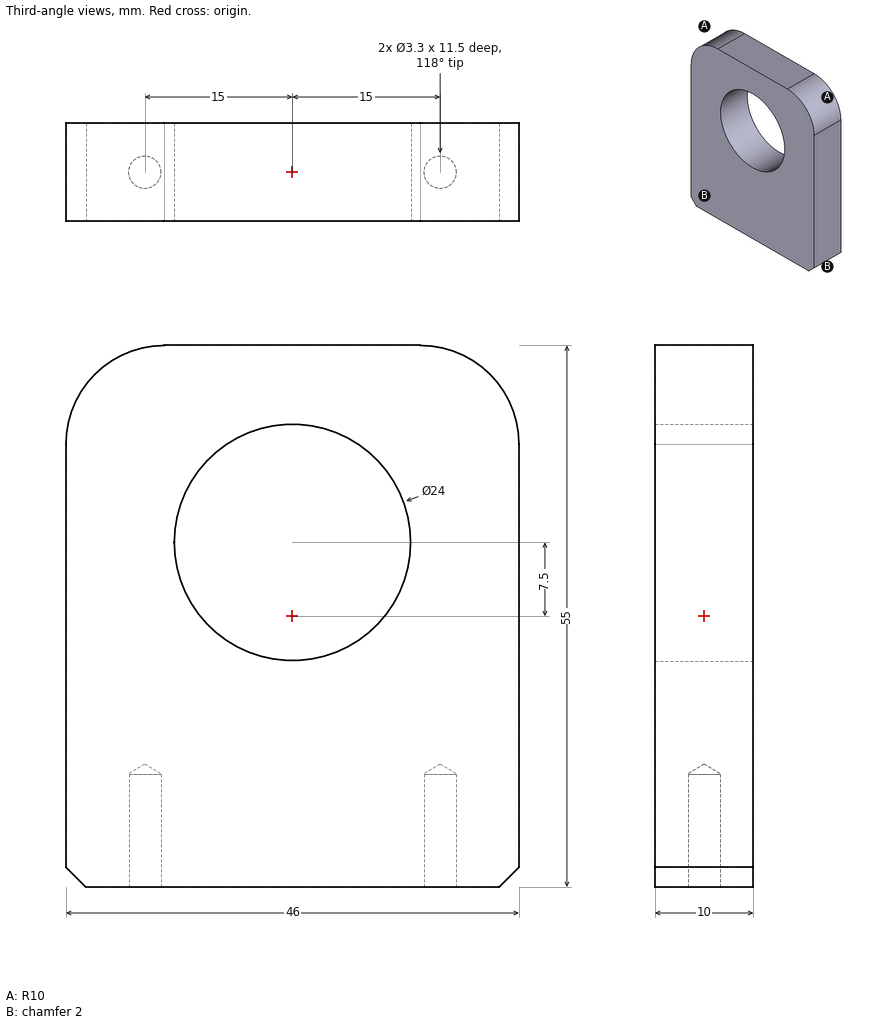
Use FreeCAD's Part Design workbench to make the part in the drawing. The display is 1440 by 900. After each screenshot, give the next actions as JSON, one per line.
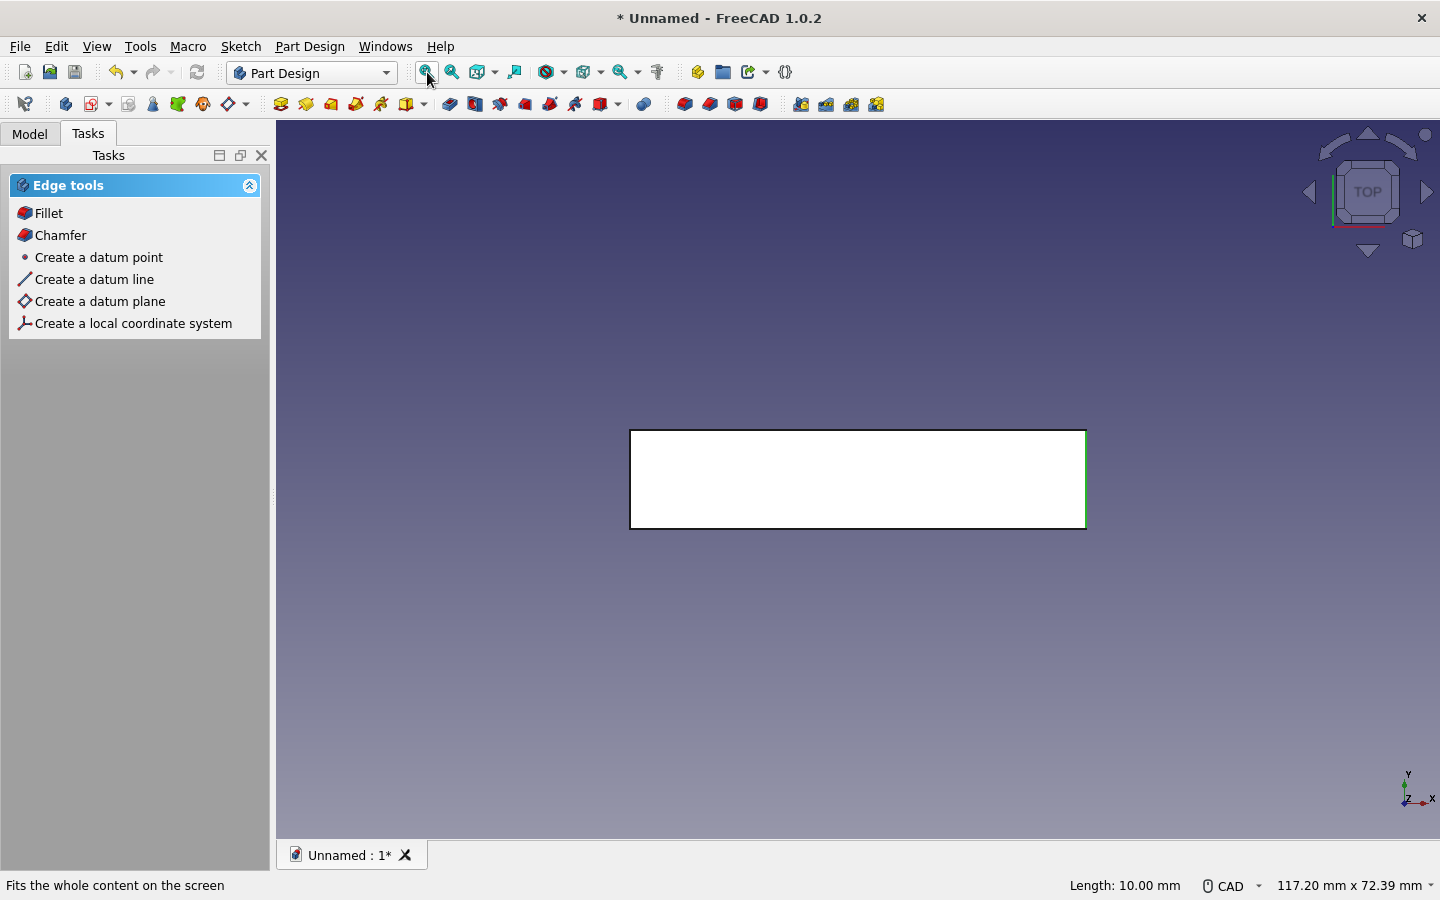
{"action": "left_click", "coordinate": [630, 478], "text": "ctrl"}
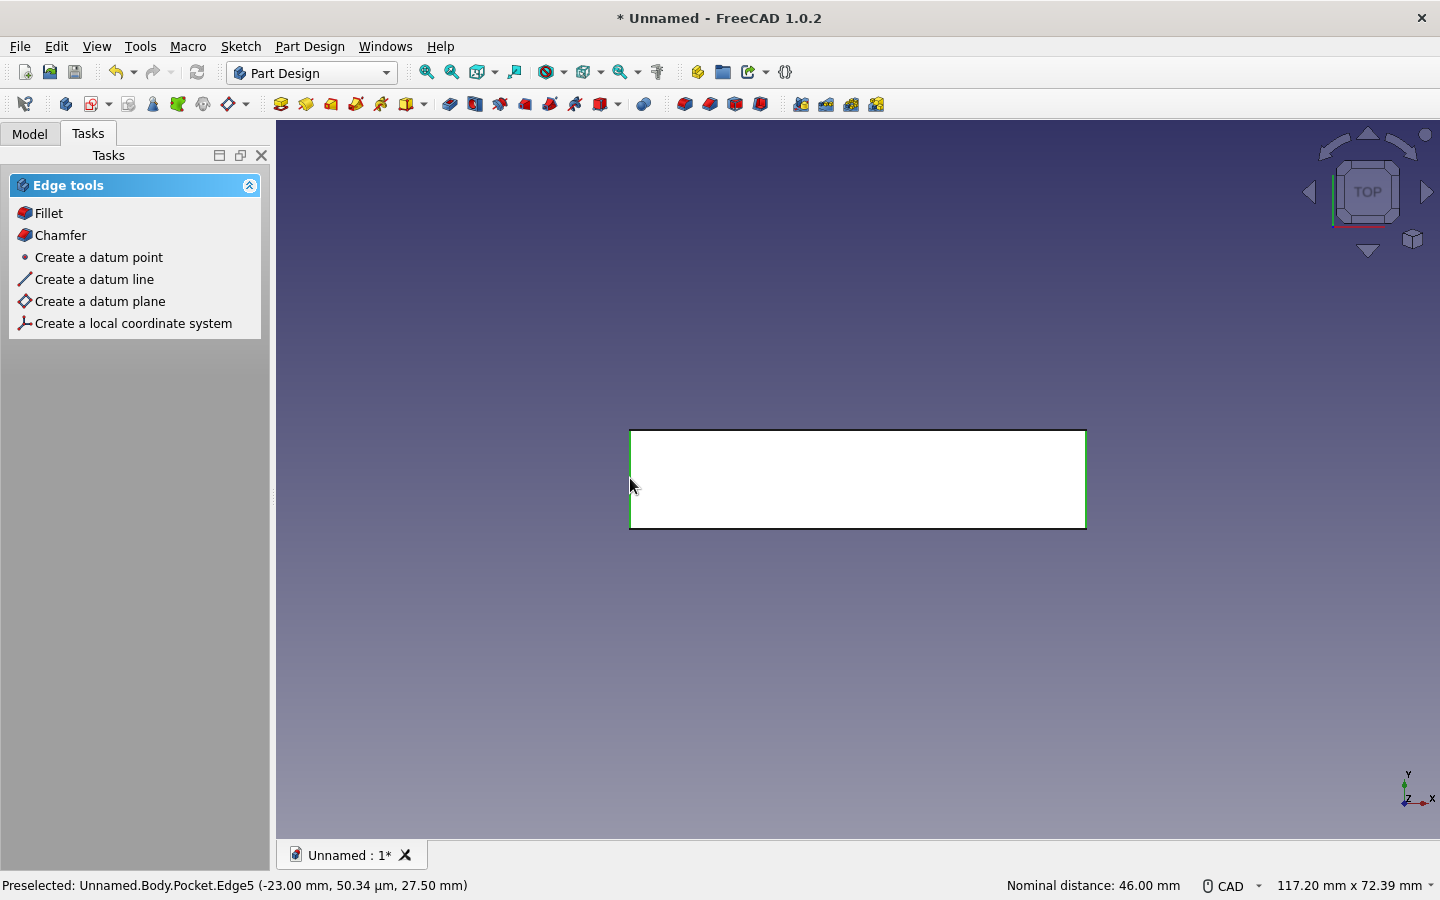
{"action": "left_click", "coordinate": [685, 104]}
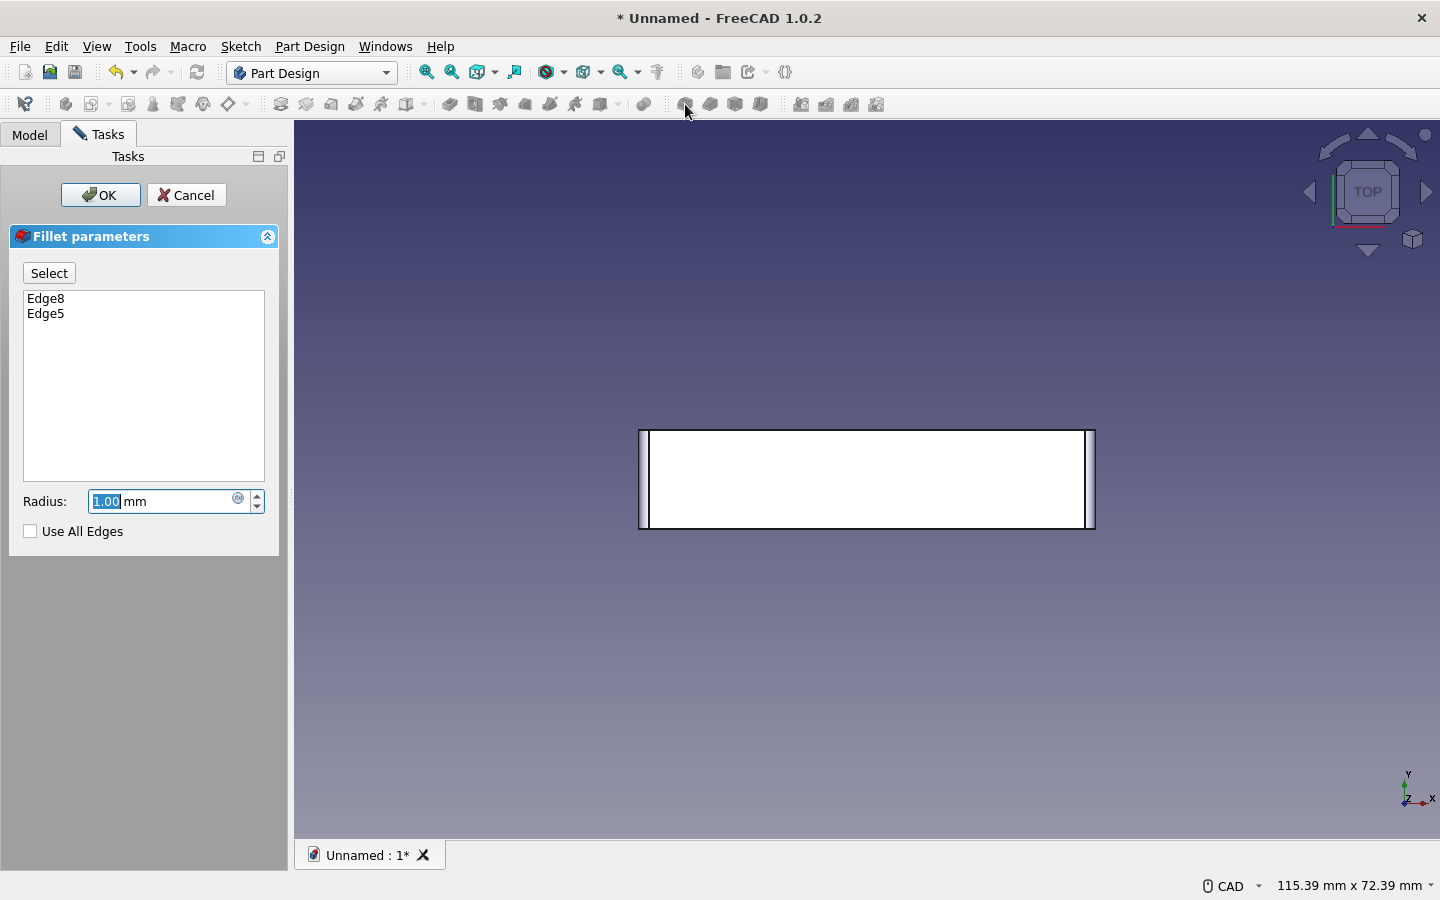
{"action": "type", "text": "10"}
{"action": "key", "text": "Tab"}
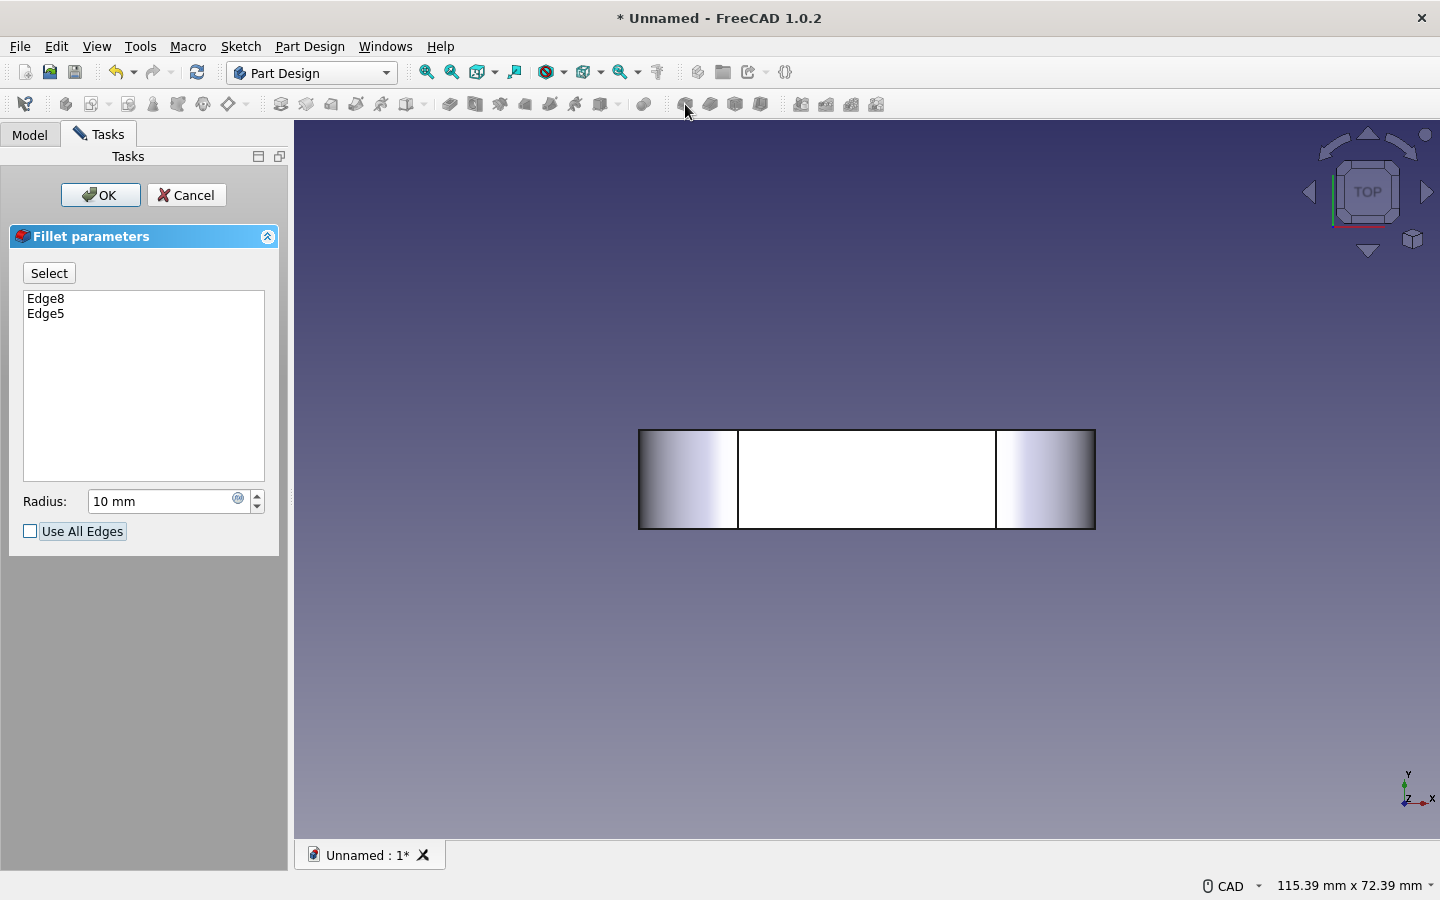
{"action": "left_click", "coordinate": [101, 195]}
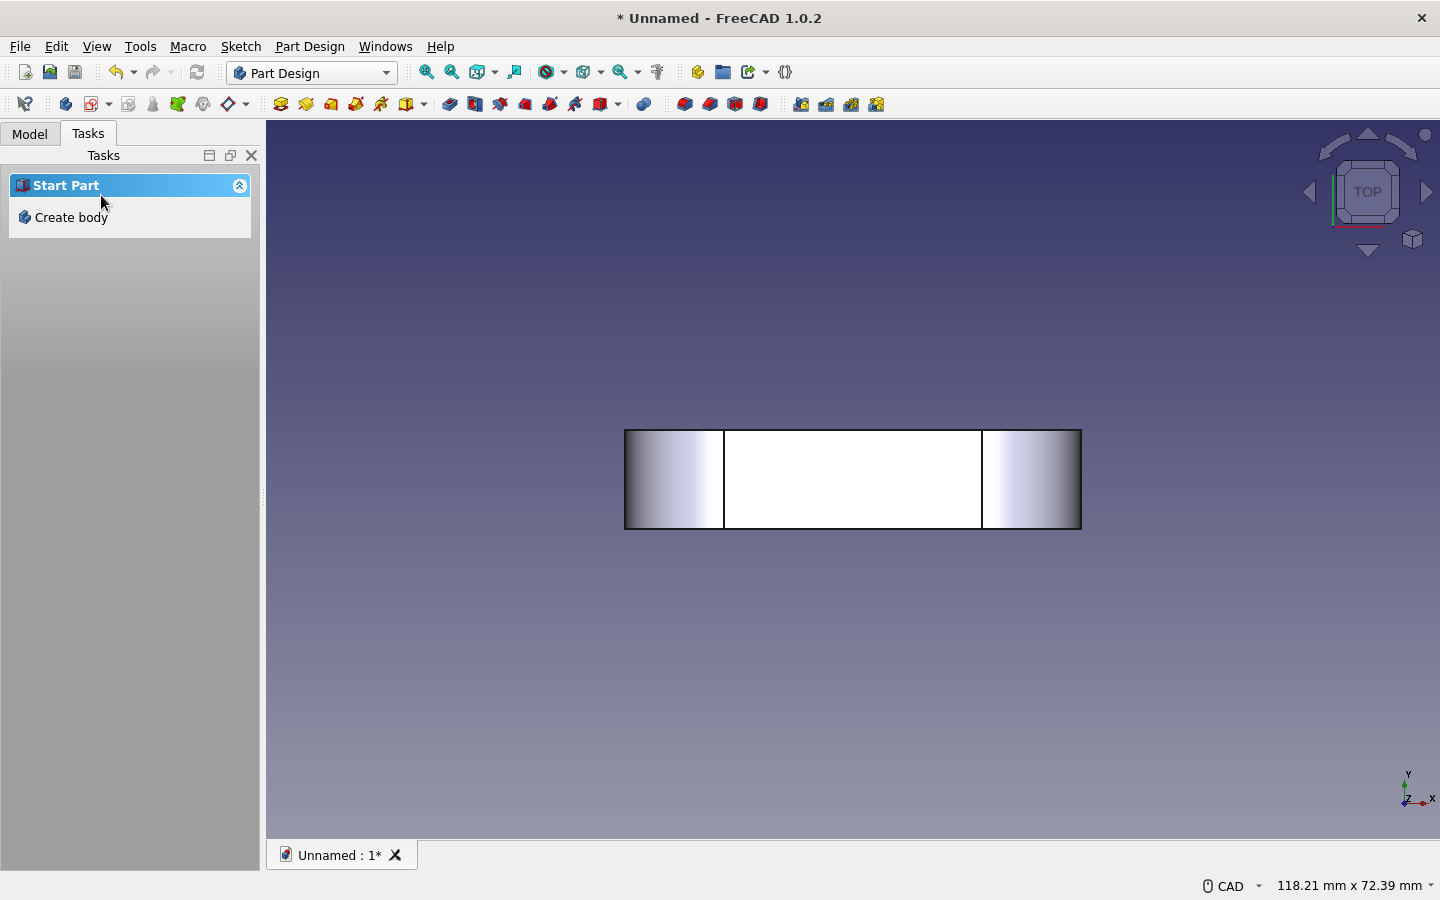
{"action": "left_click", "coordinate": [427, 72]}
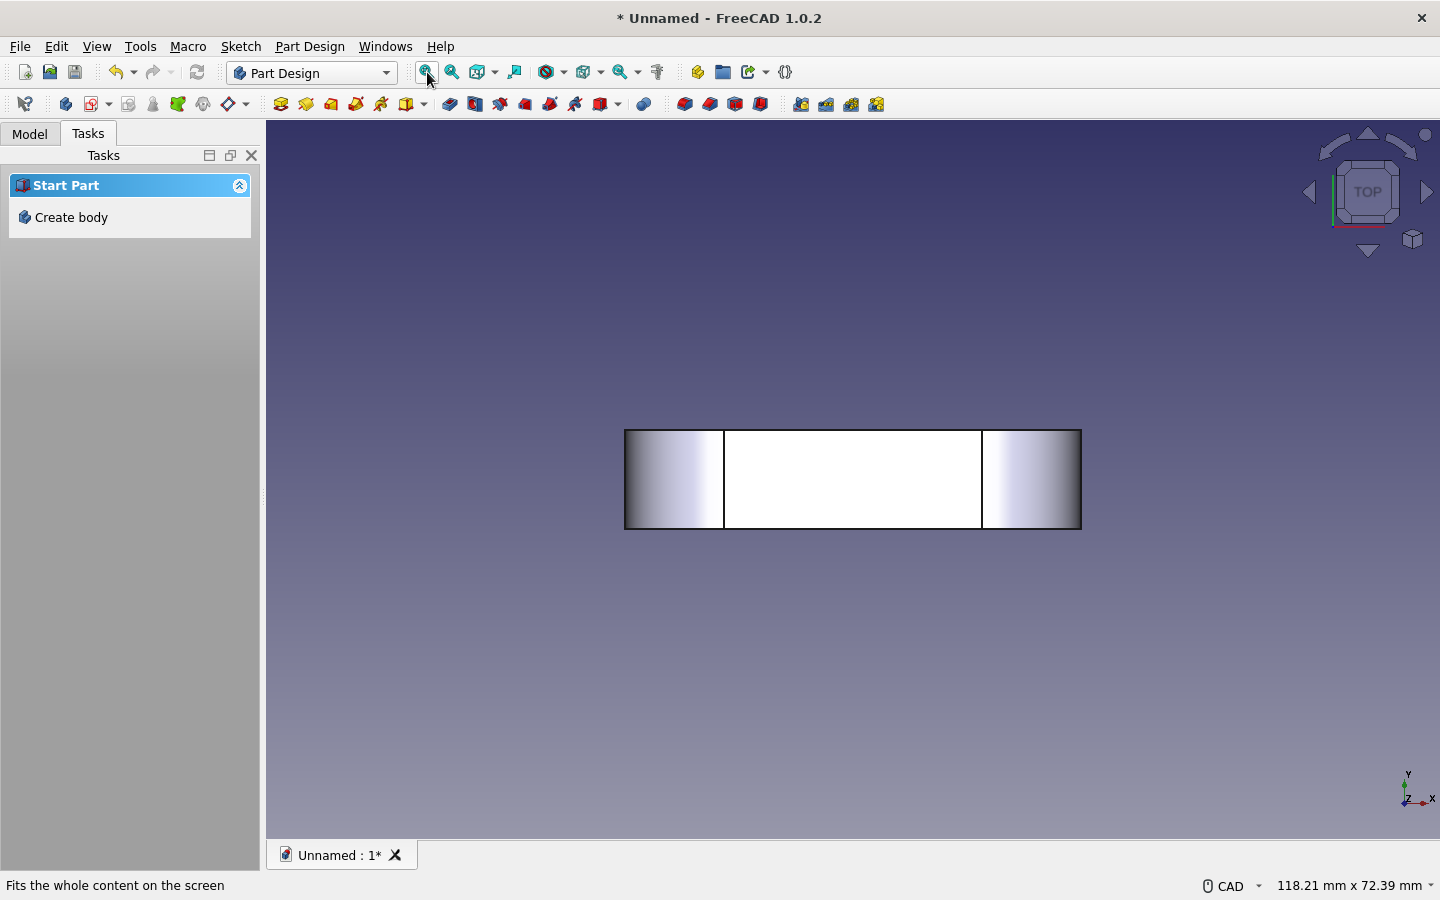
{"action": "key", "text": "5"}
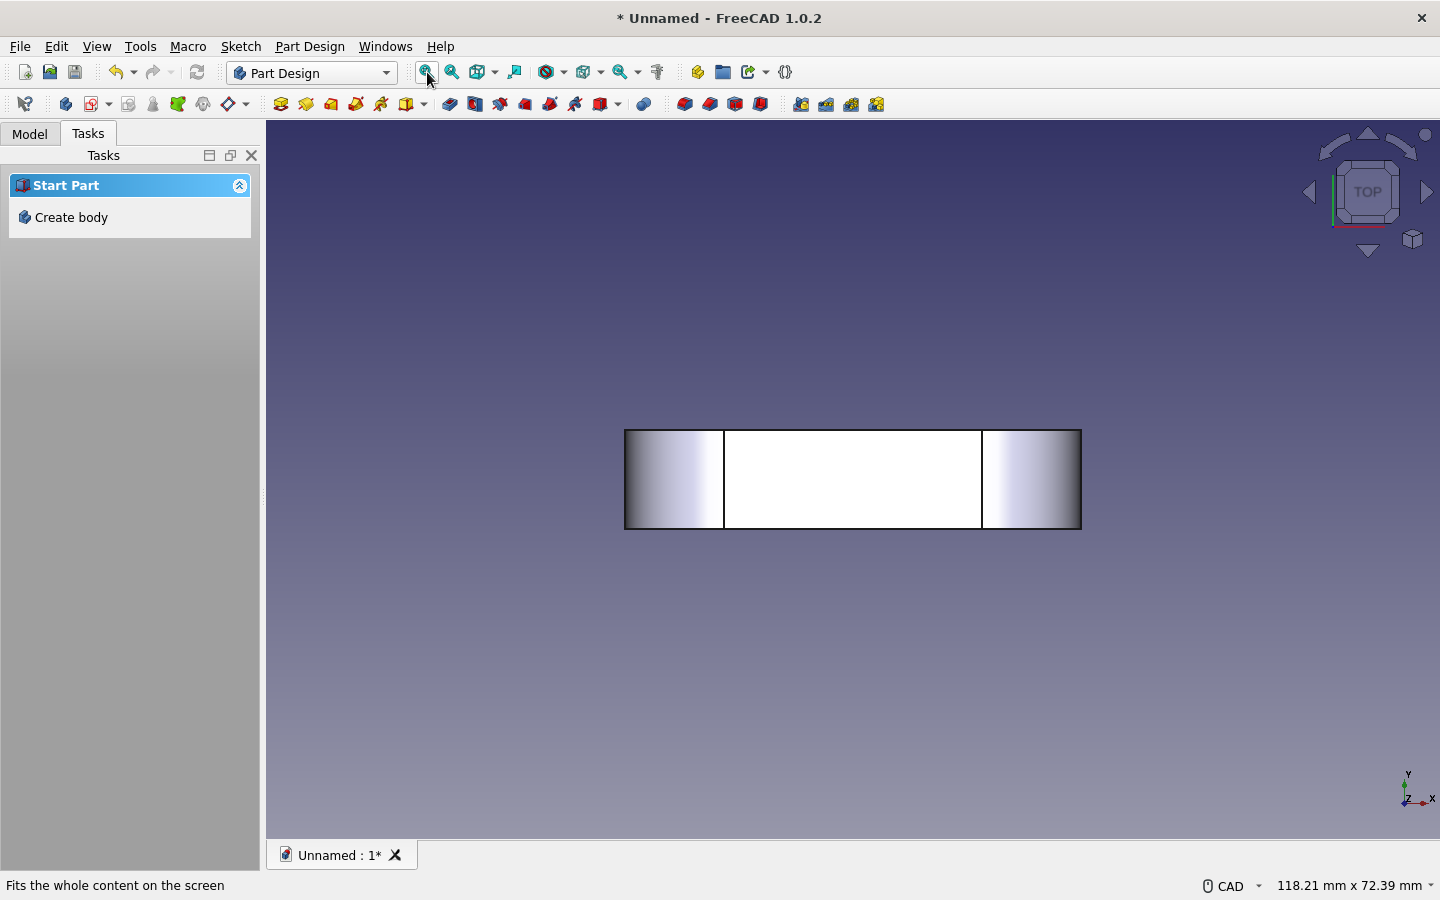
{"action": "left_click", "coordinate": [427, 72]}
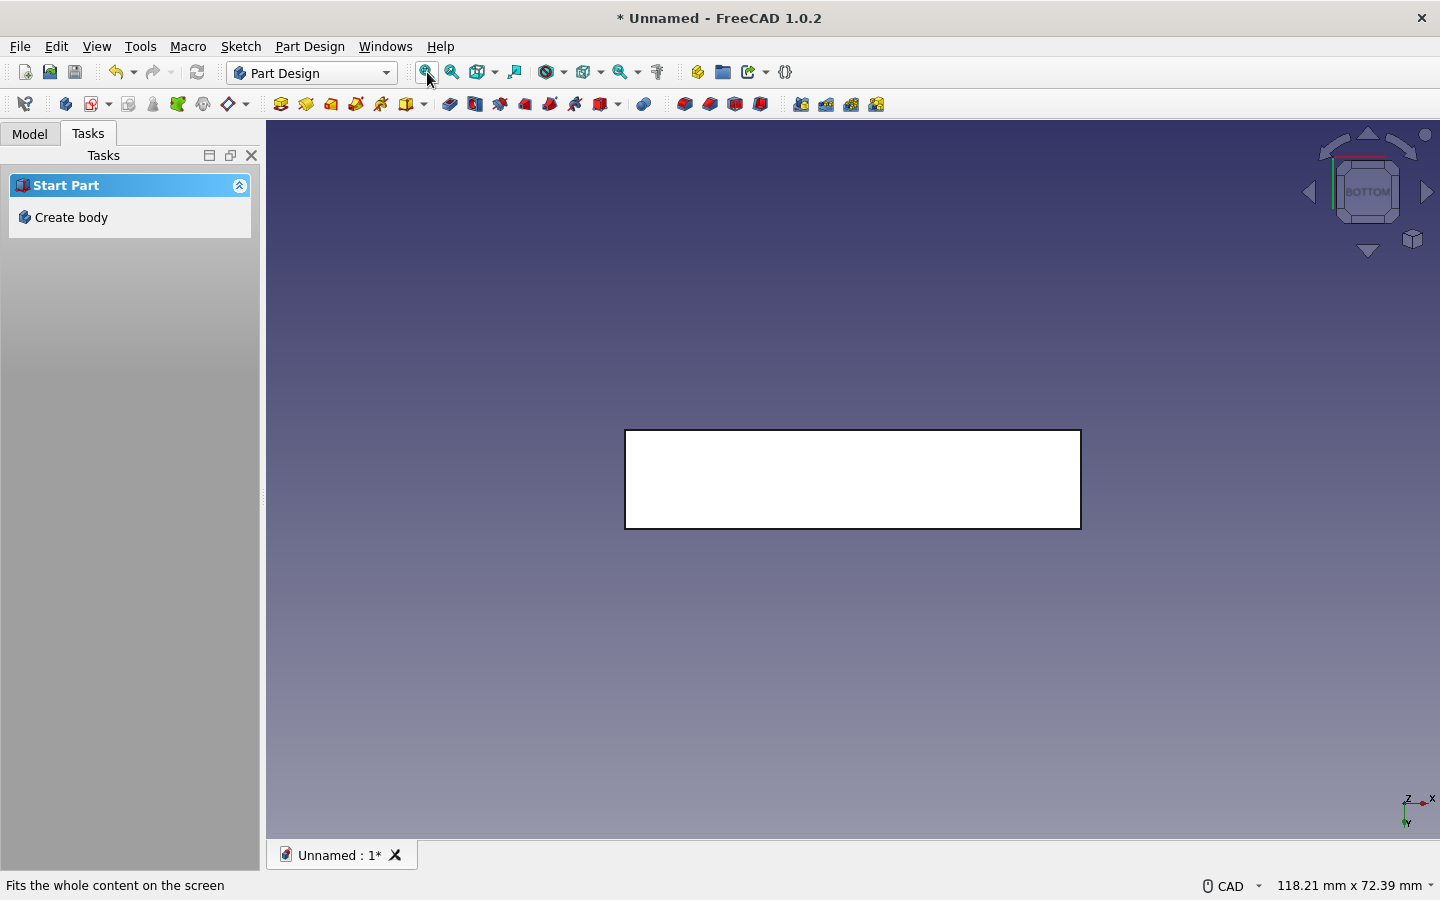
{"action": "left_click", "coordinate": [984, 478]}